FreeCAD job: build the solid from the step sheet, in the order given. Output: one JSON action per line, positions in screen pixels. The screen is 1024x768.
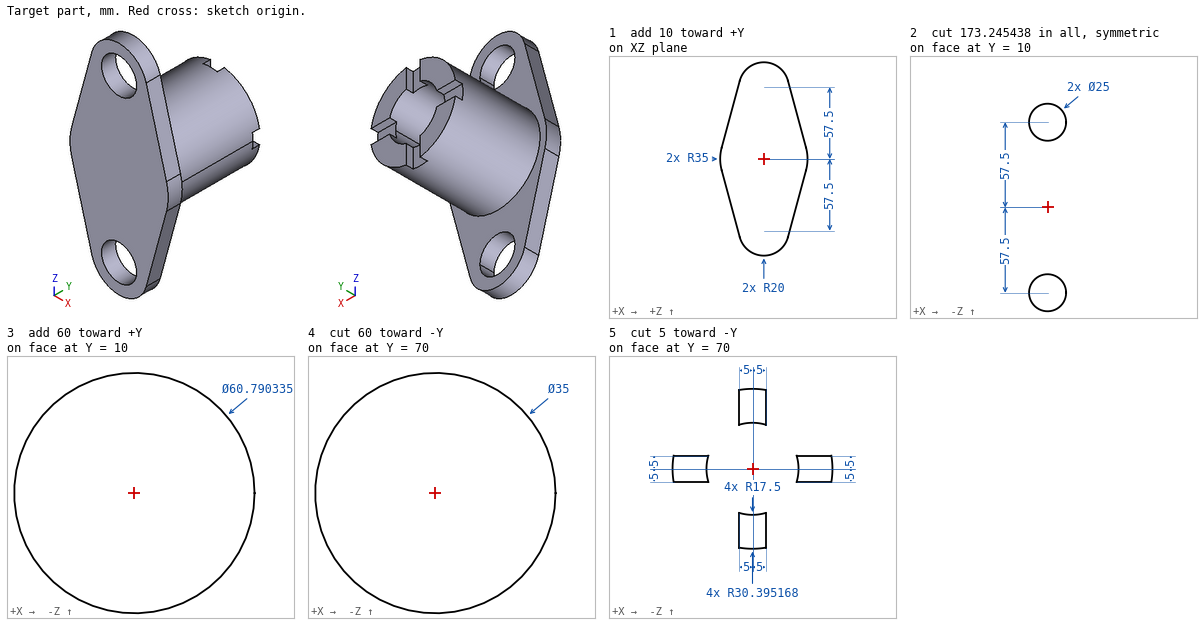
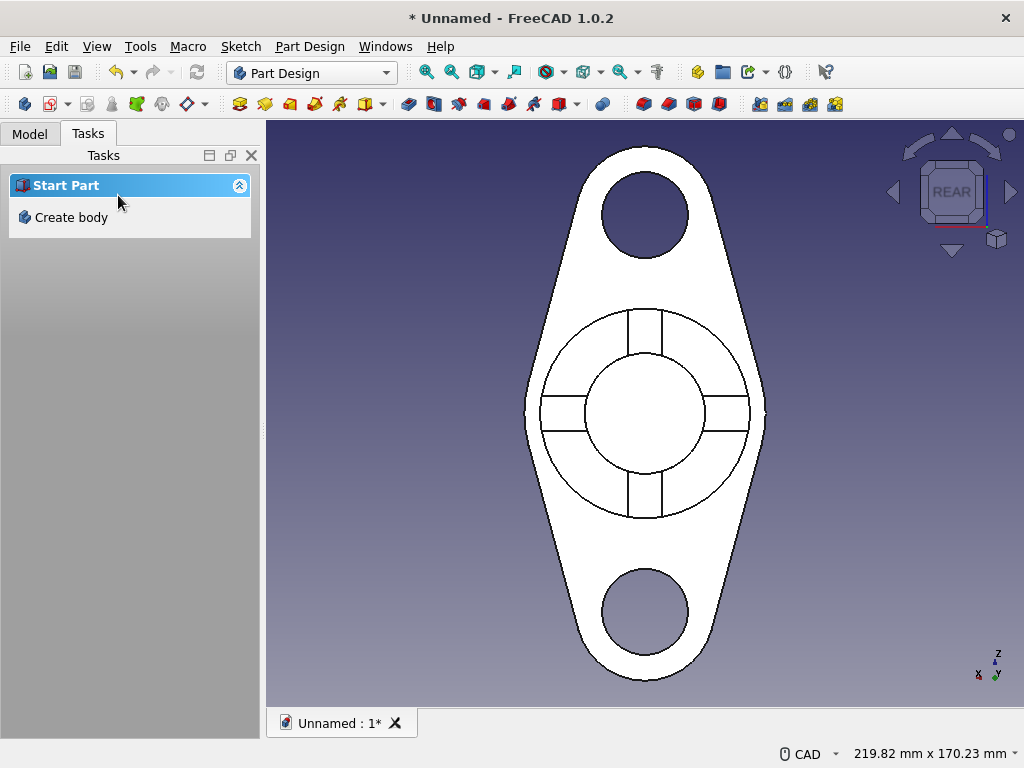
{"action": "key", "text": "0"}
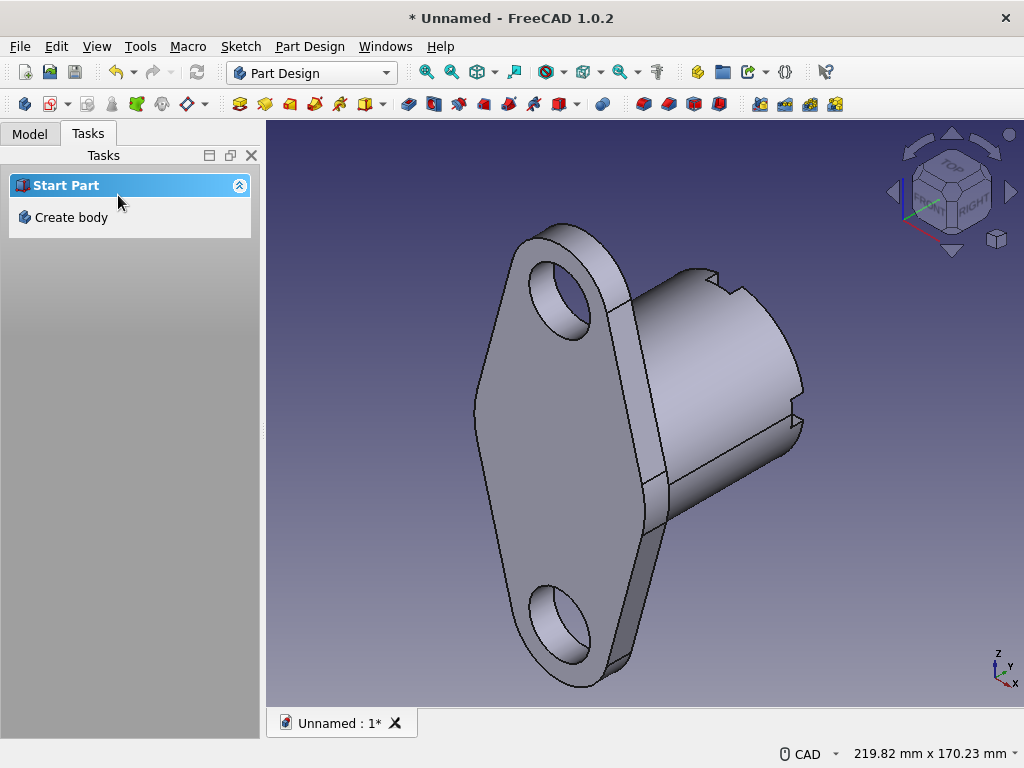
{"action": "left_click", "coordinate": [427, 72]}